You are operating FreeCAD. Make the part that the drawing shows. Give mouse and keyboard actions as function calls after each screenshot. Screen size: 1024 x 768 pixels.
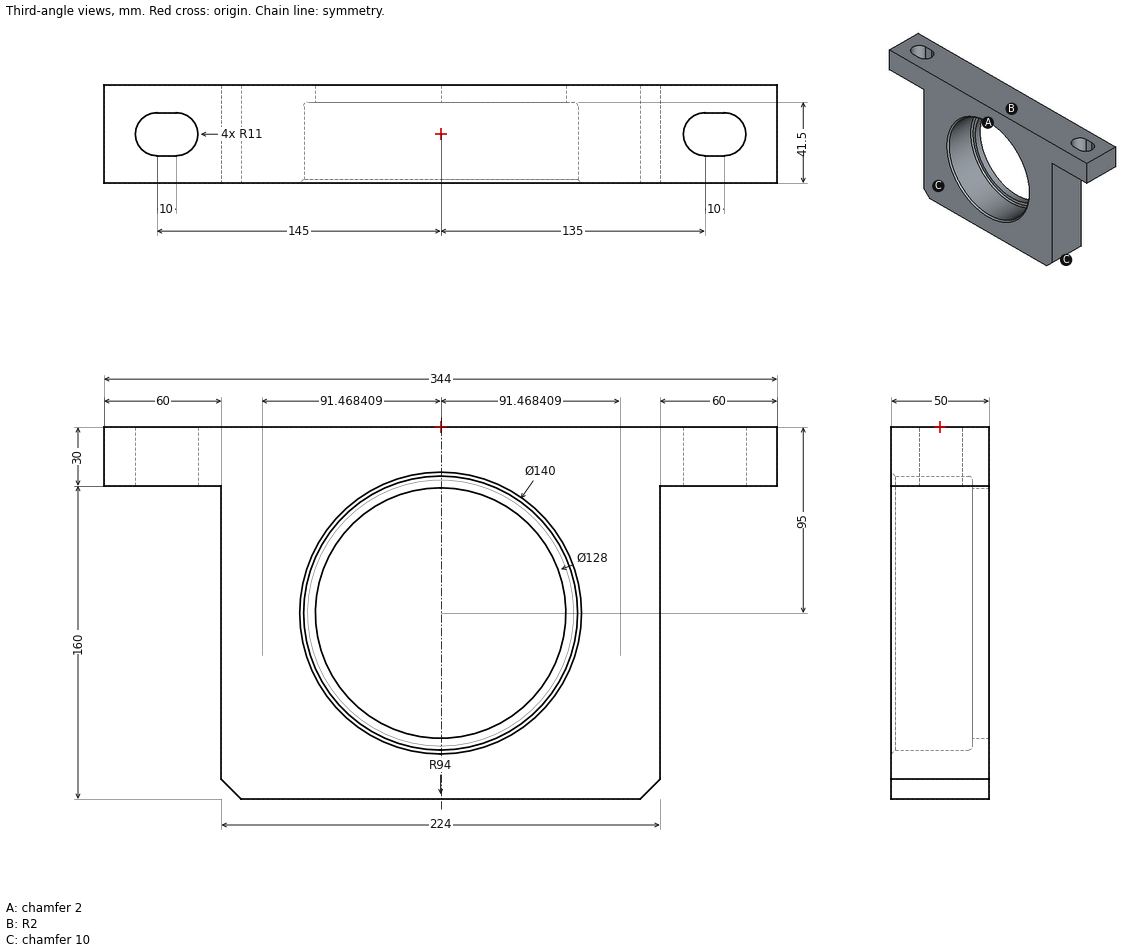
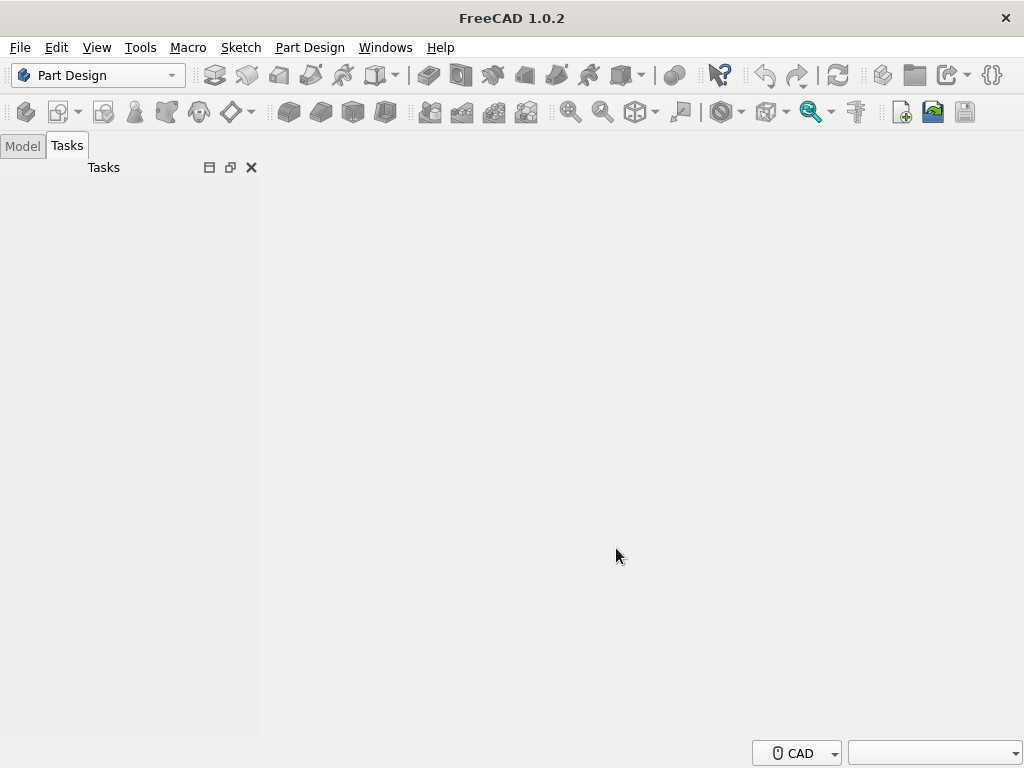
key(ctrl+n)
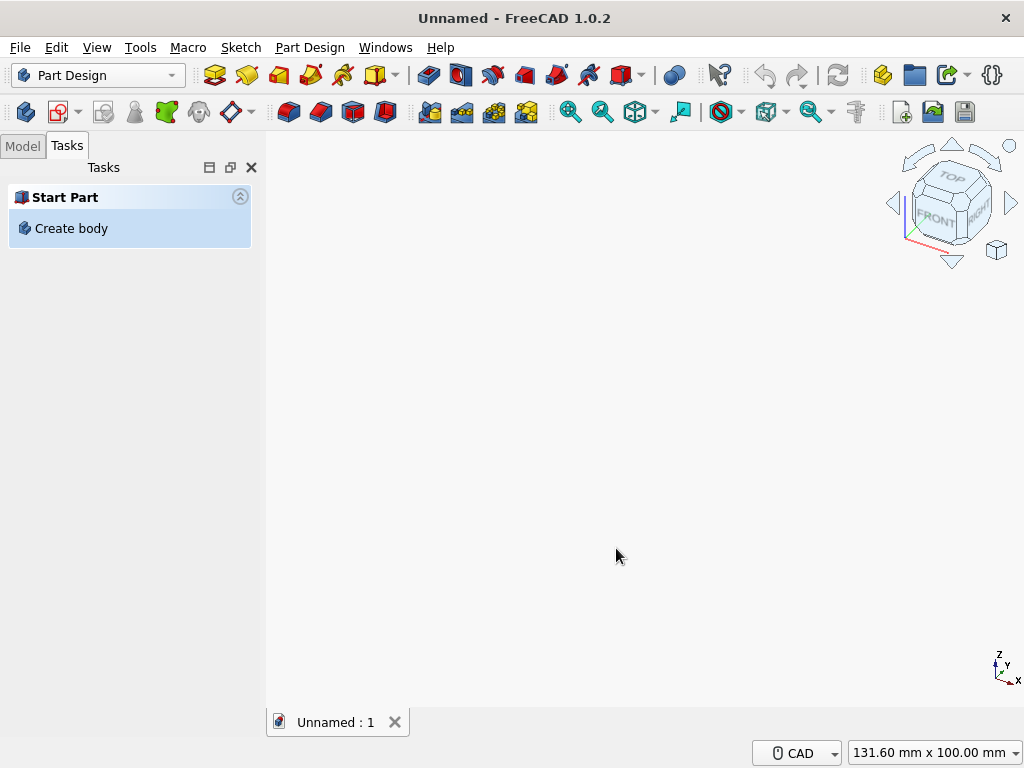
click(58, 112)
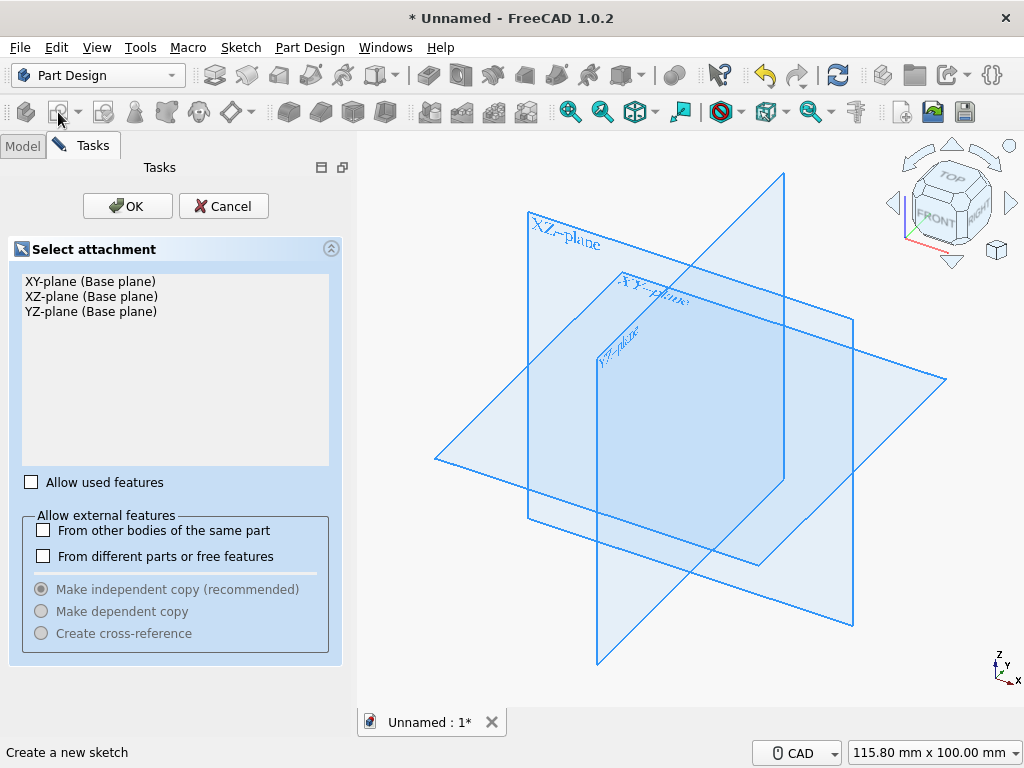
click(82, 296)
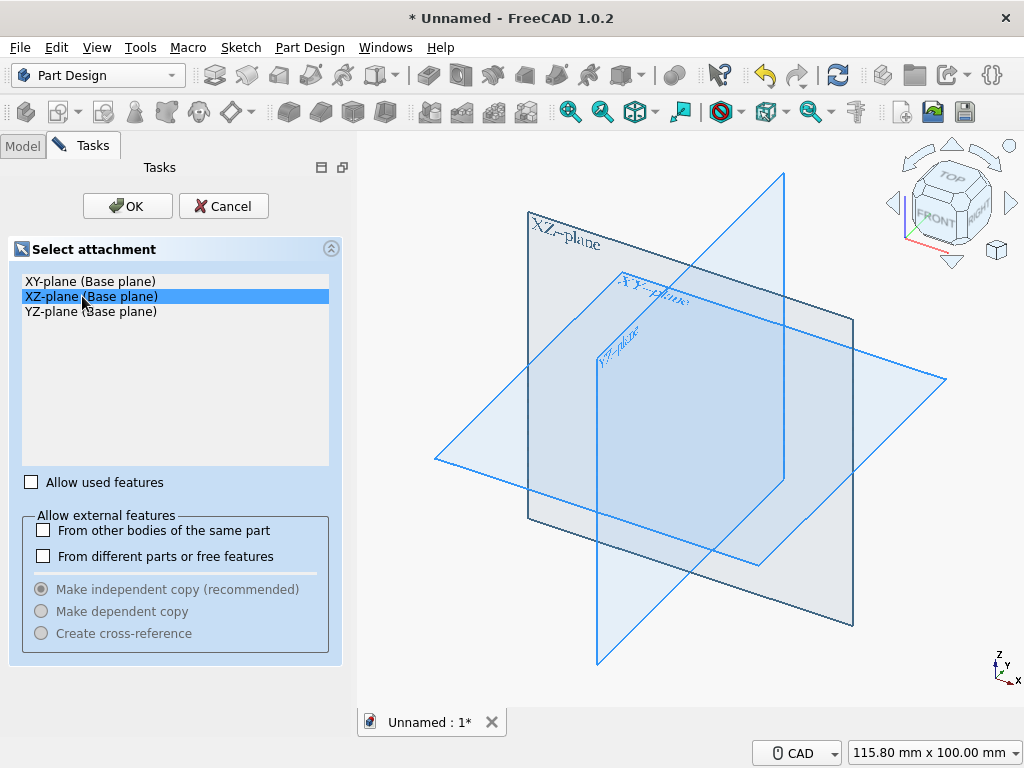
click(128, 206)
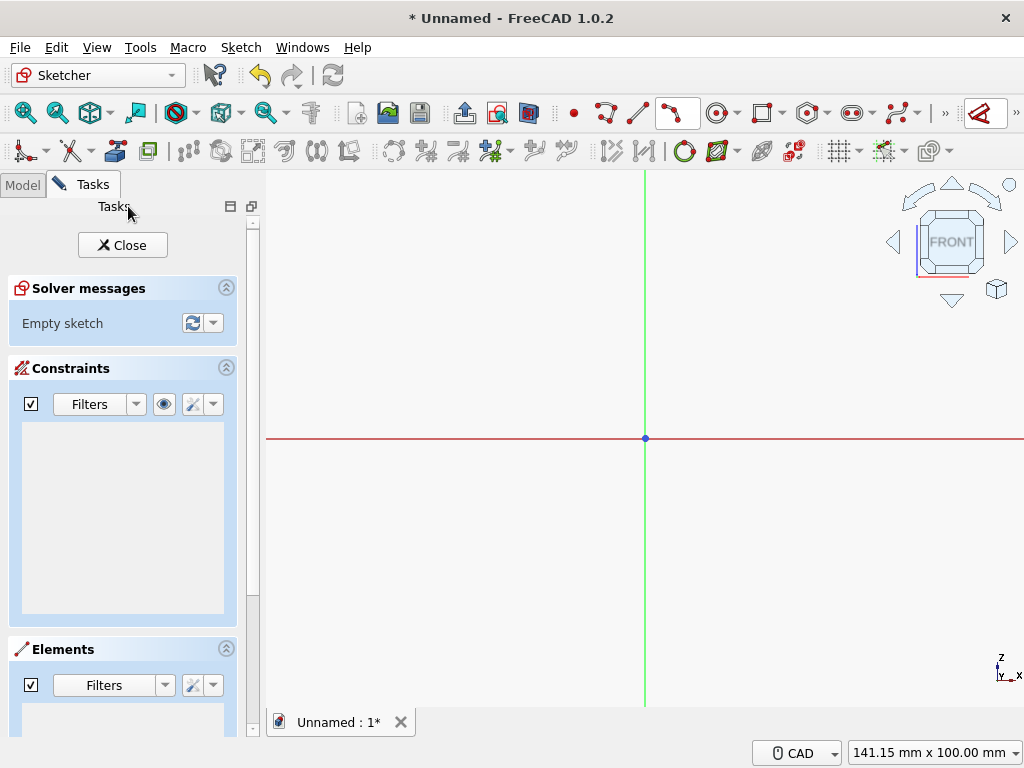
scroll(559, 310, down, 8)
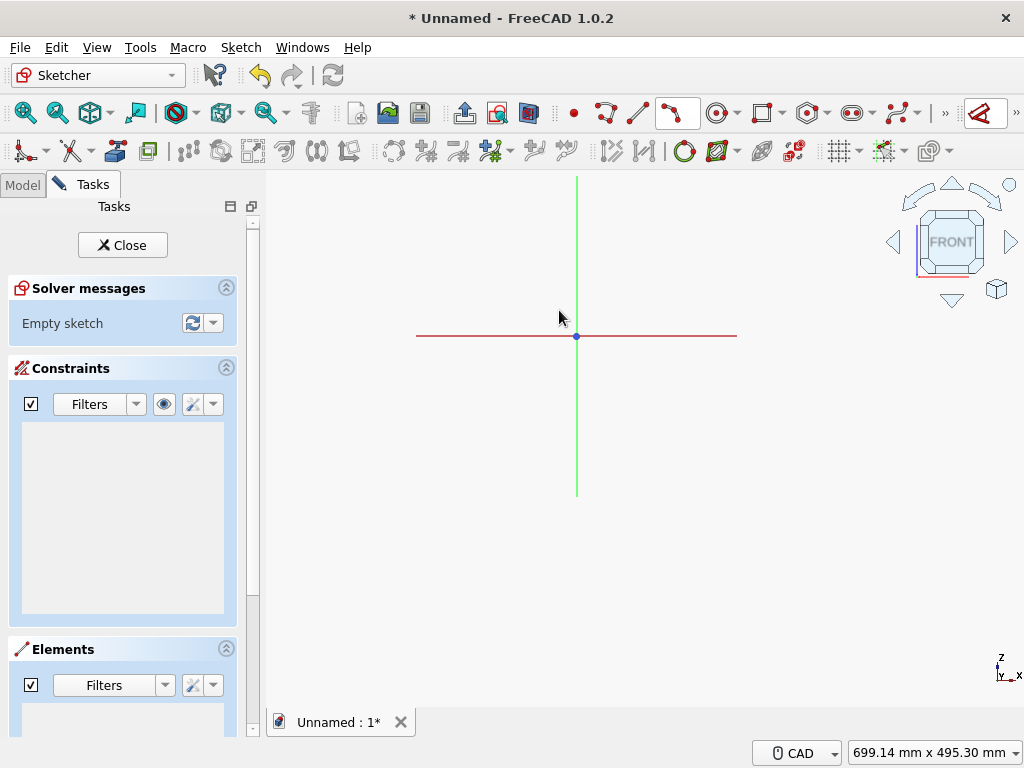
key(g)
key(m)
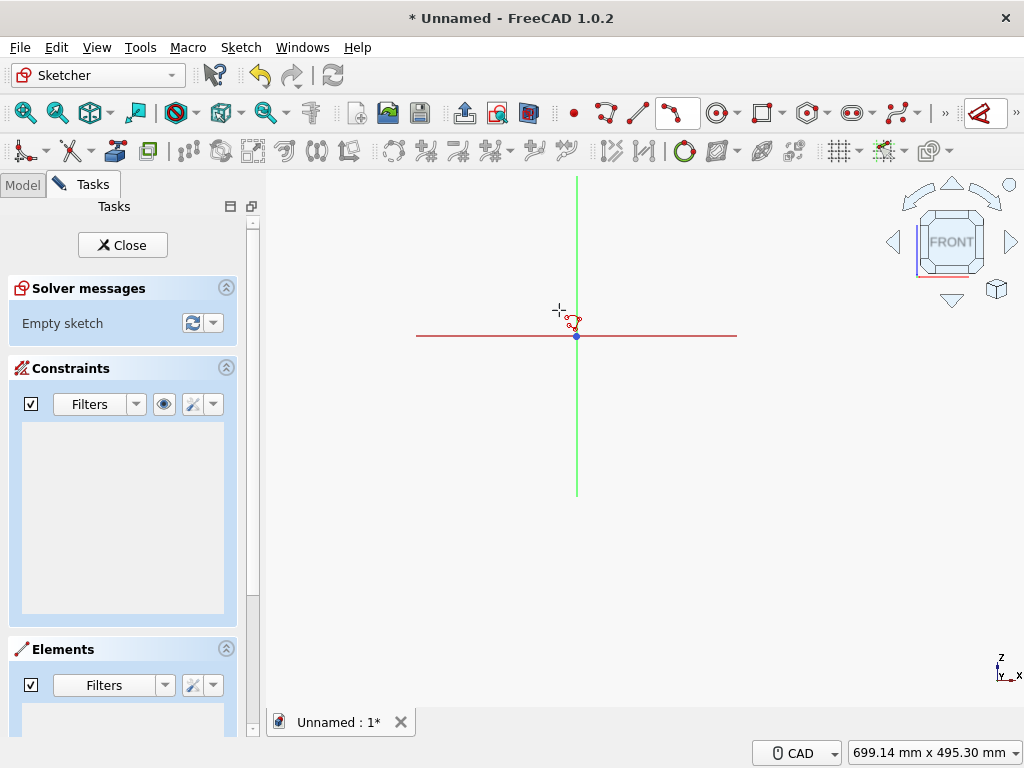
click(478, 463)
click(455, 369)
click(390, 369)
click(390, 336)
click(763, 345)
click(763, 369)
click(698, 369)
click(676, 463)
right_click(676, 463)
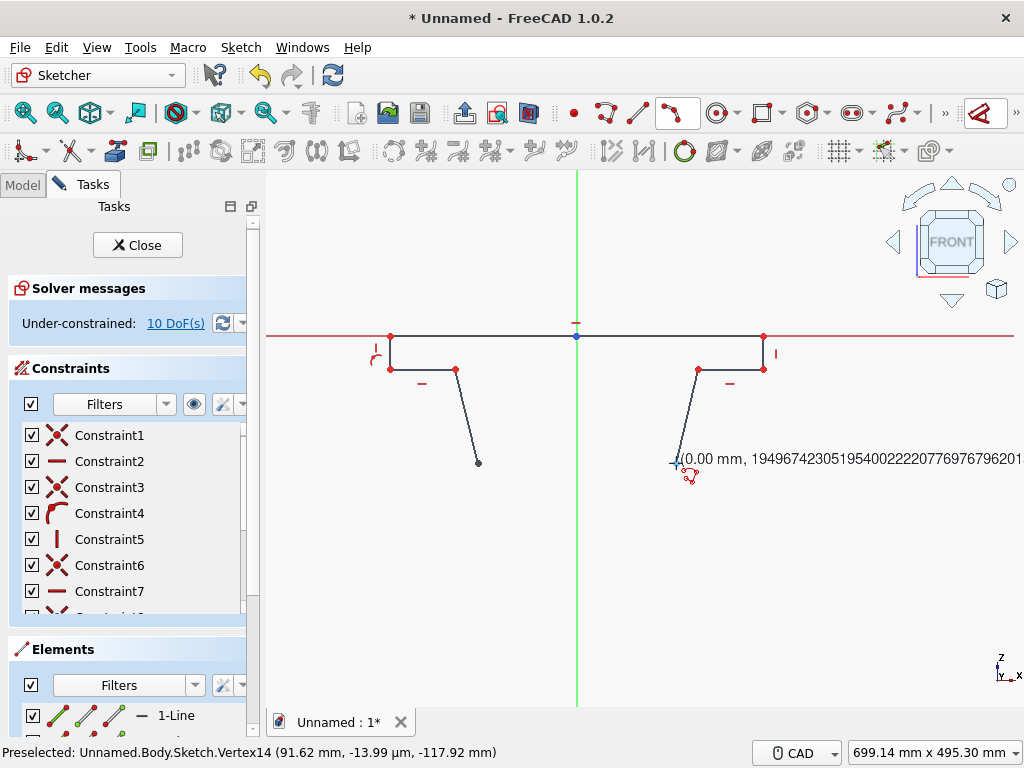
key(g)
key(3)
key(a)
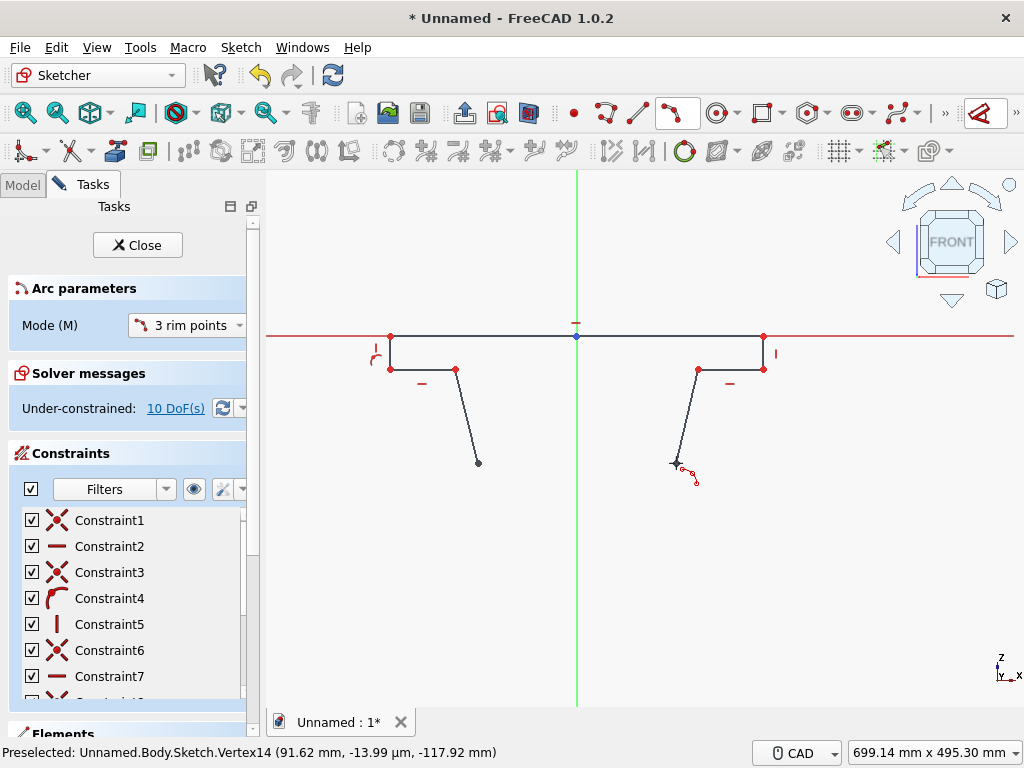
click(676, 464)
click(478, 464)
click(550, 537)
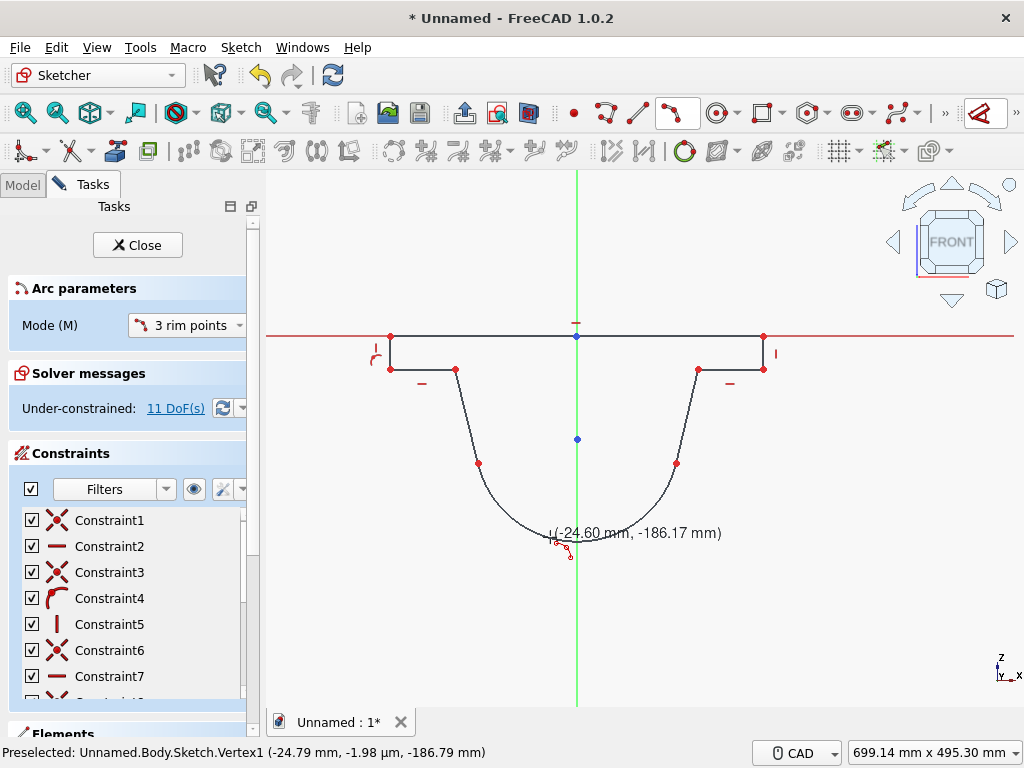
key(g)
key(c)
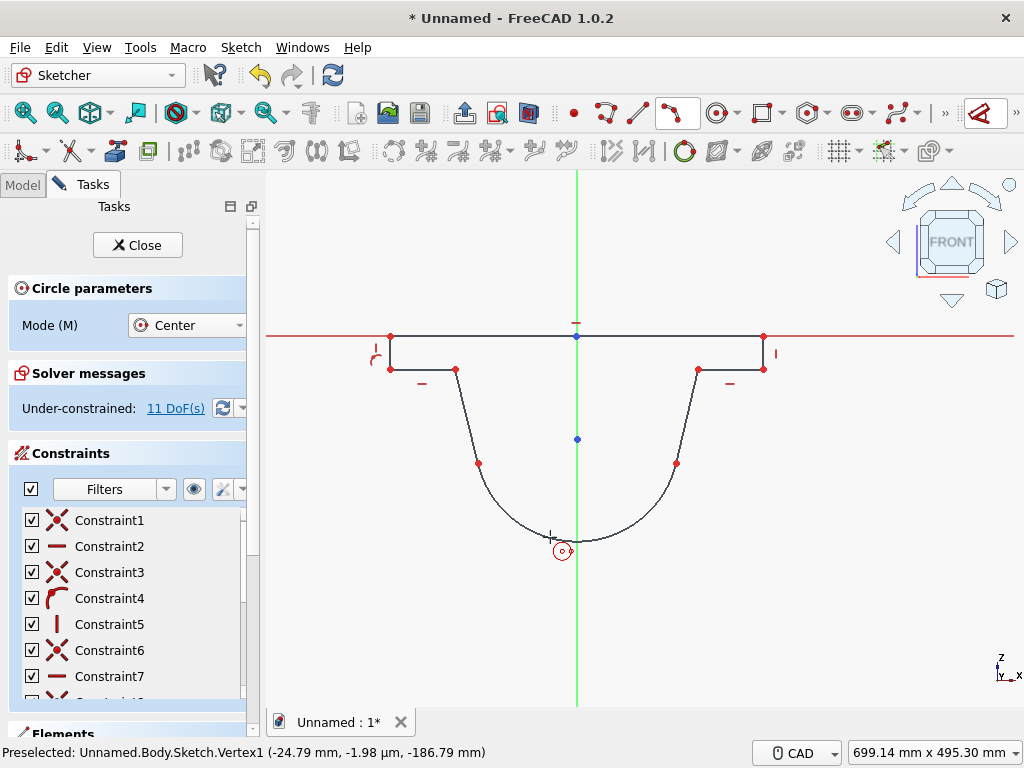
click(577, 439)
move(626, 390)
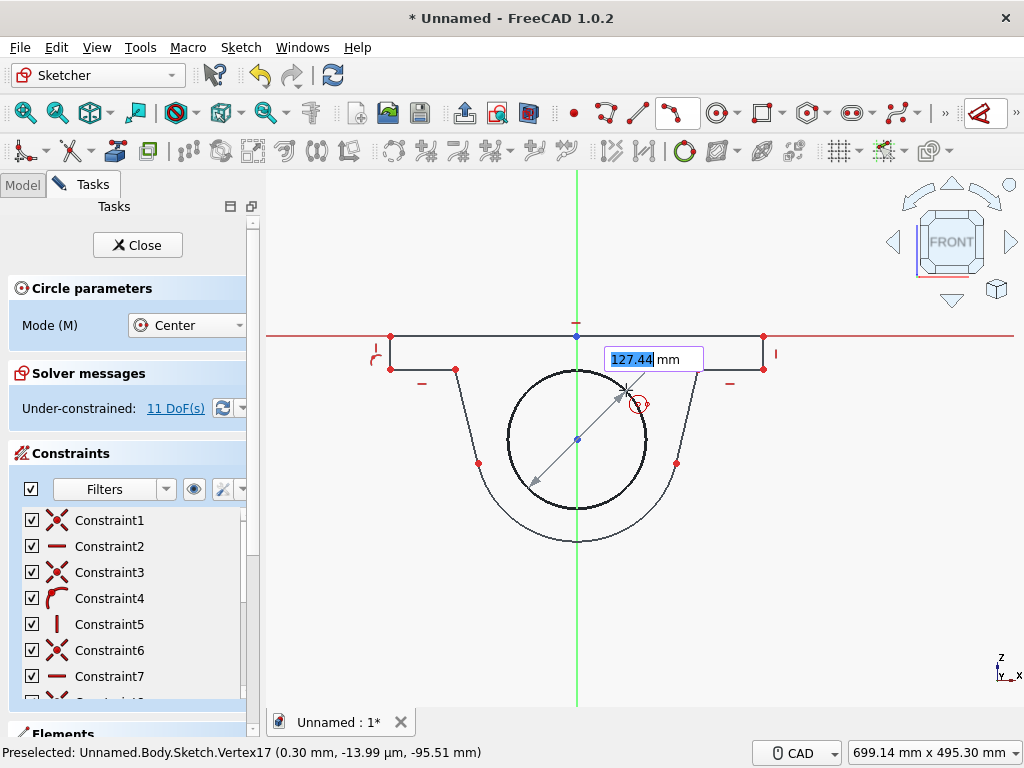
text(128)
key(Return)
key(Escape)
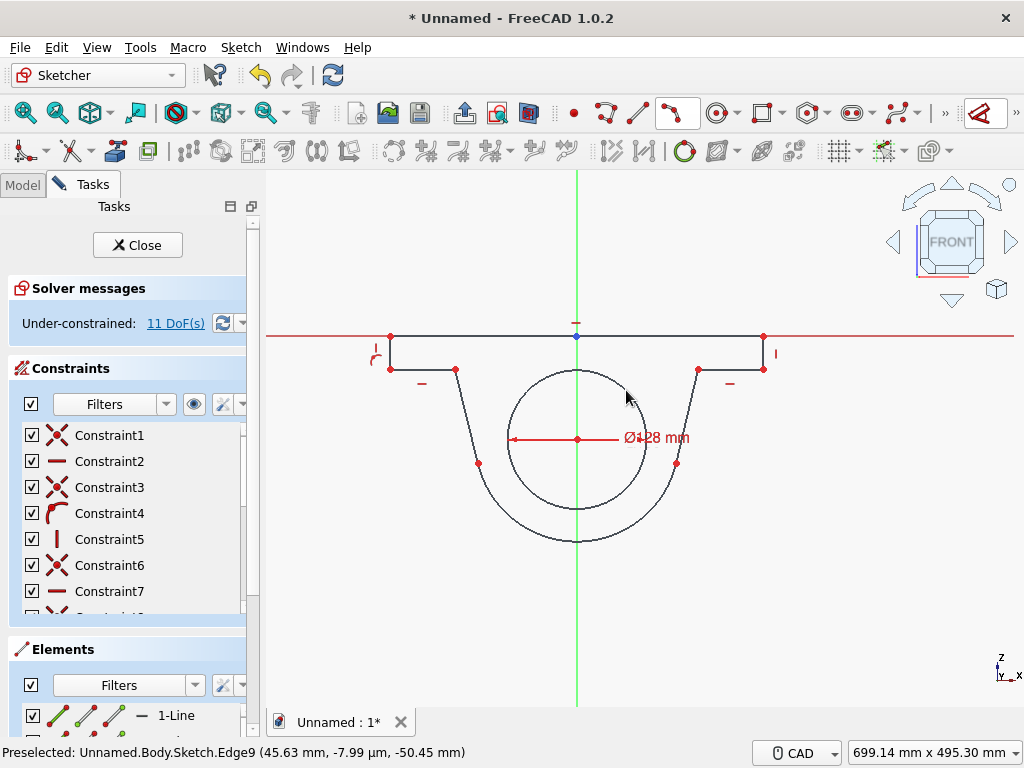
click(577, 440)